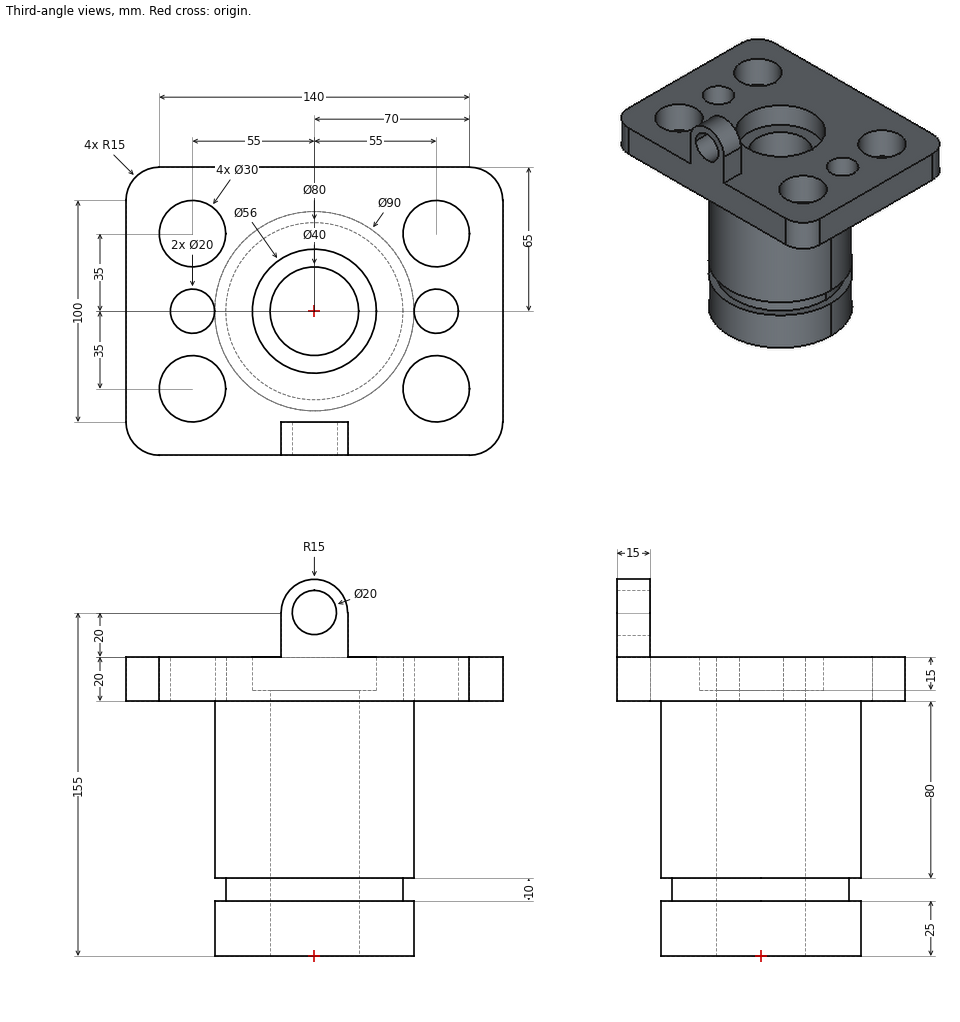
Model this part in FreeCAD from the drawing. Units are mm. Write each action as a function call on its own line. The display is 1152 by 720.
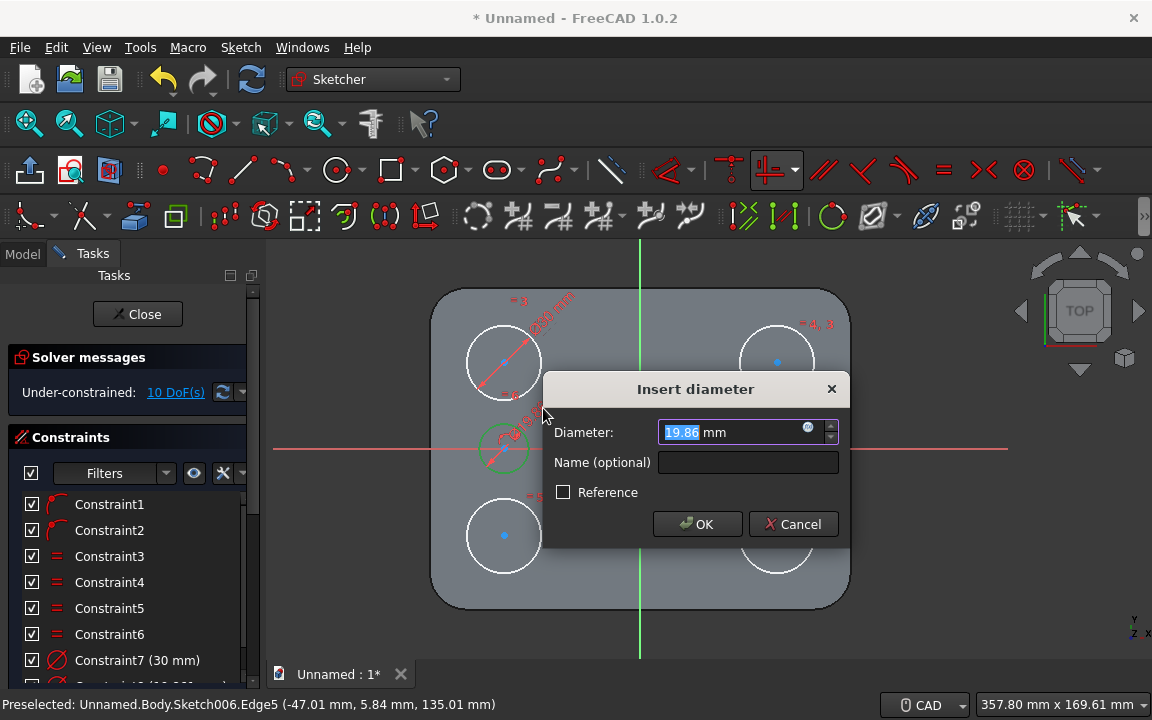
text(20)
key(Return)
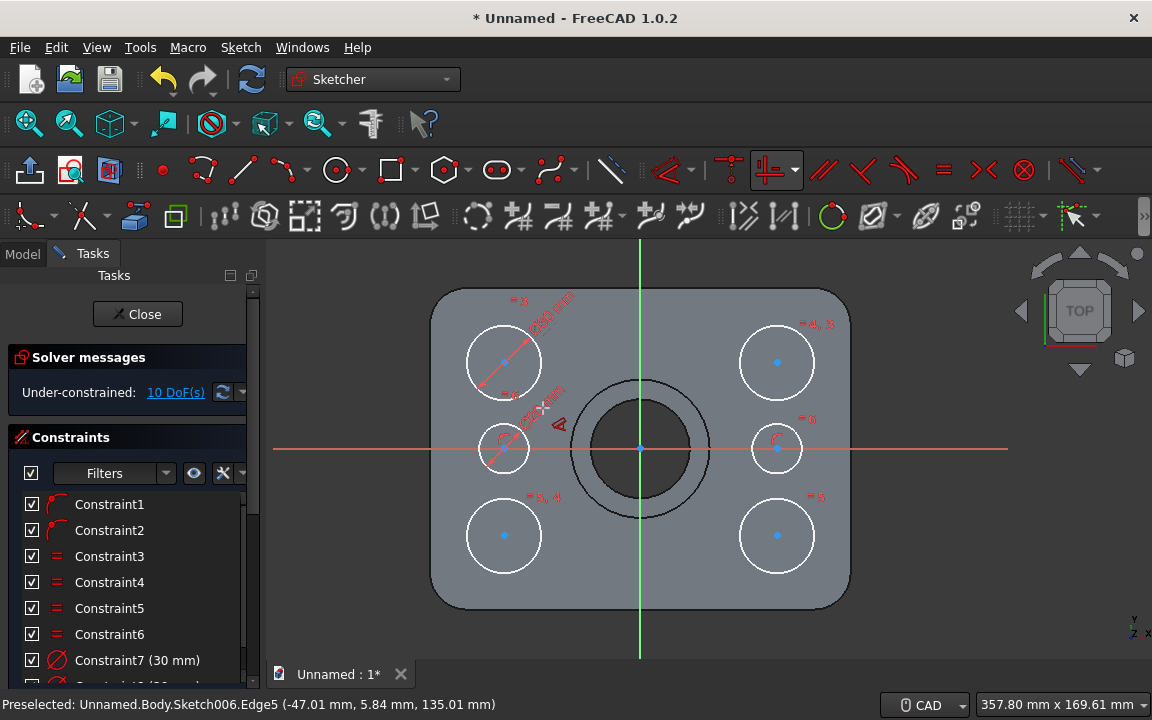
click(504, 363)
click(572, 483)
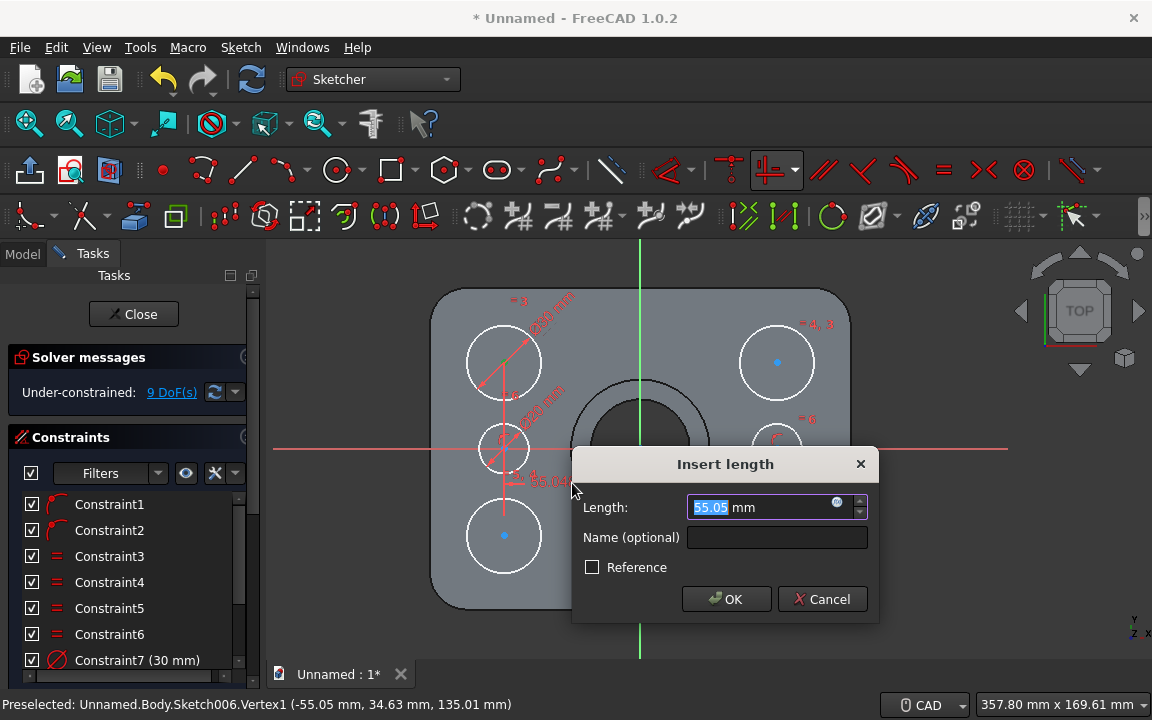
text(55)
key(Return)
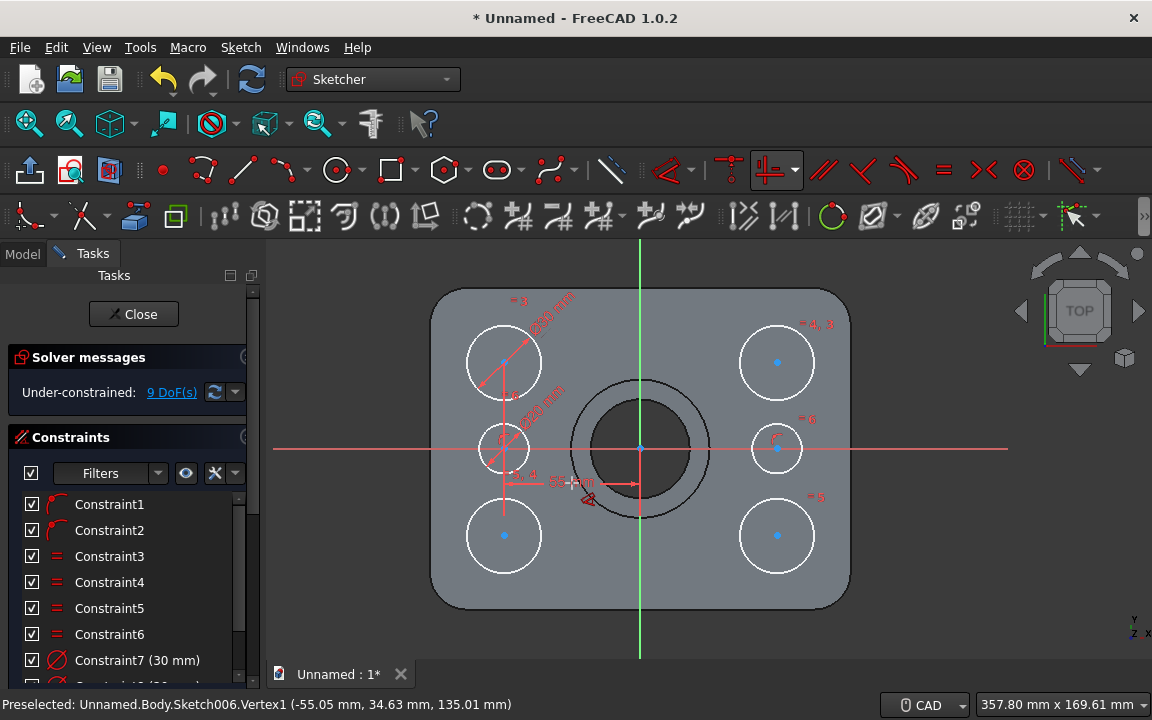
click(504, 363)
click(470, 406)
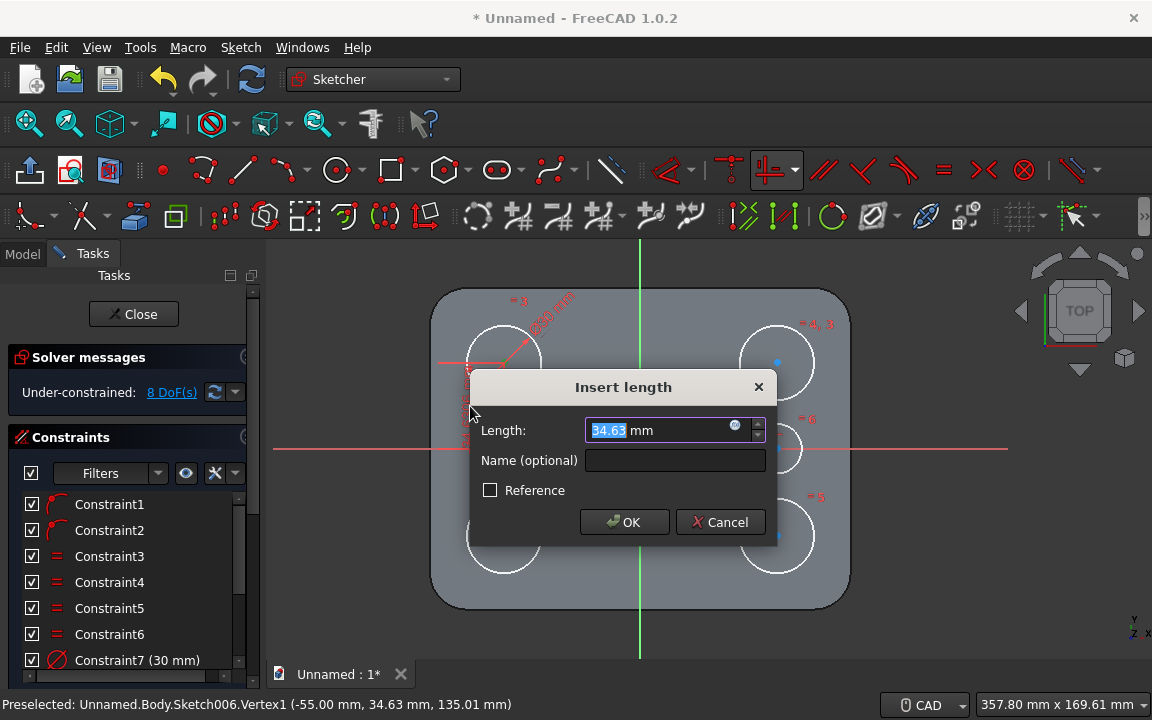
text(35)
key(Return)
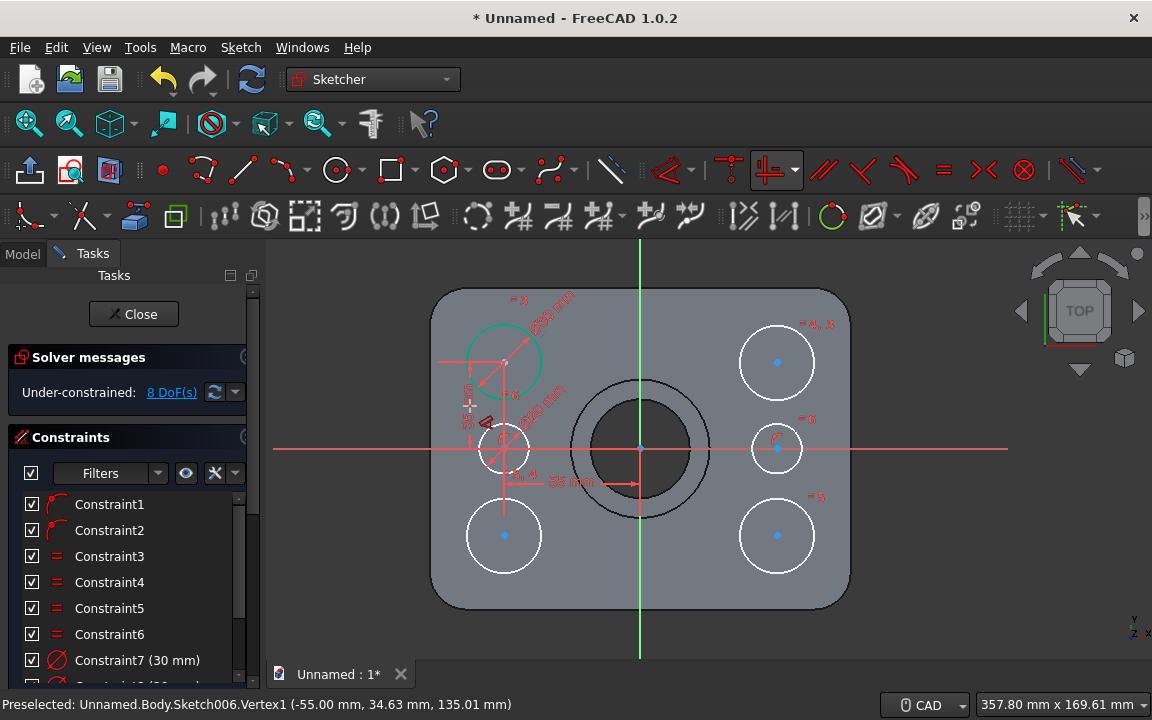
click(777, 363)
click(709, 329)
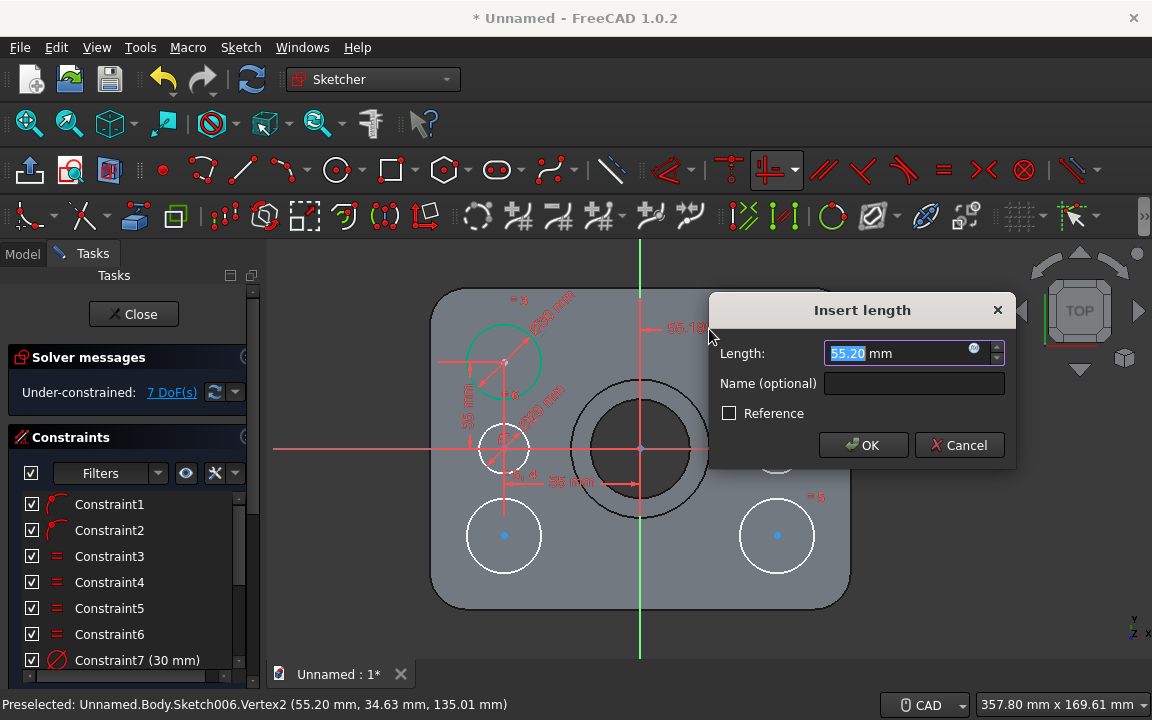
text(55)
key(Return)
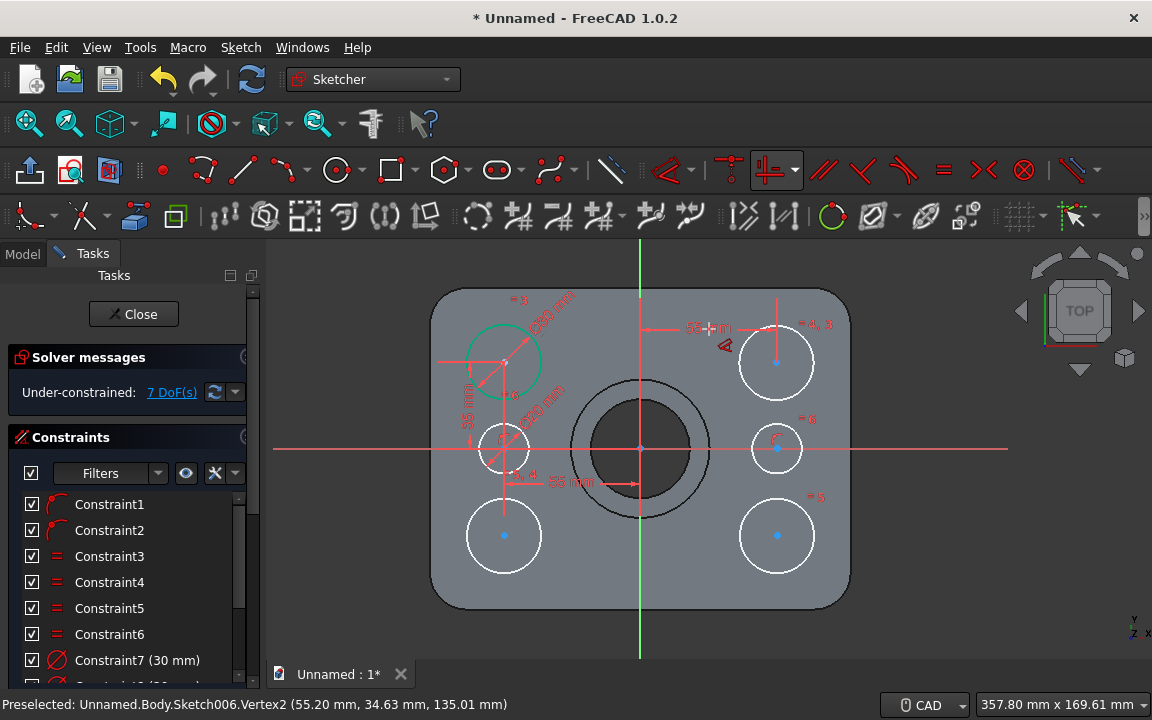
click(777, 363)
click(811, 406)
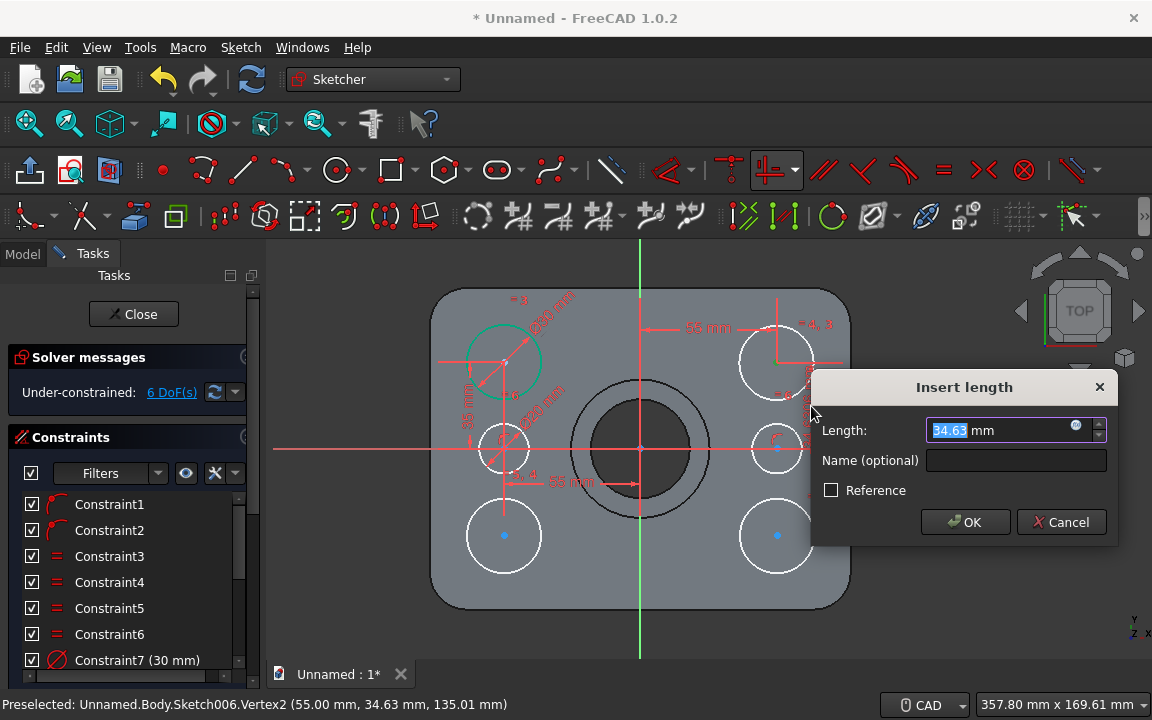
text(35)
key(Return)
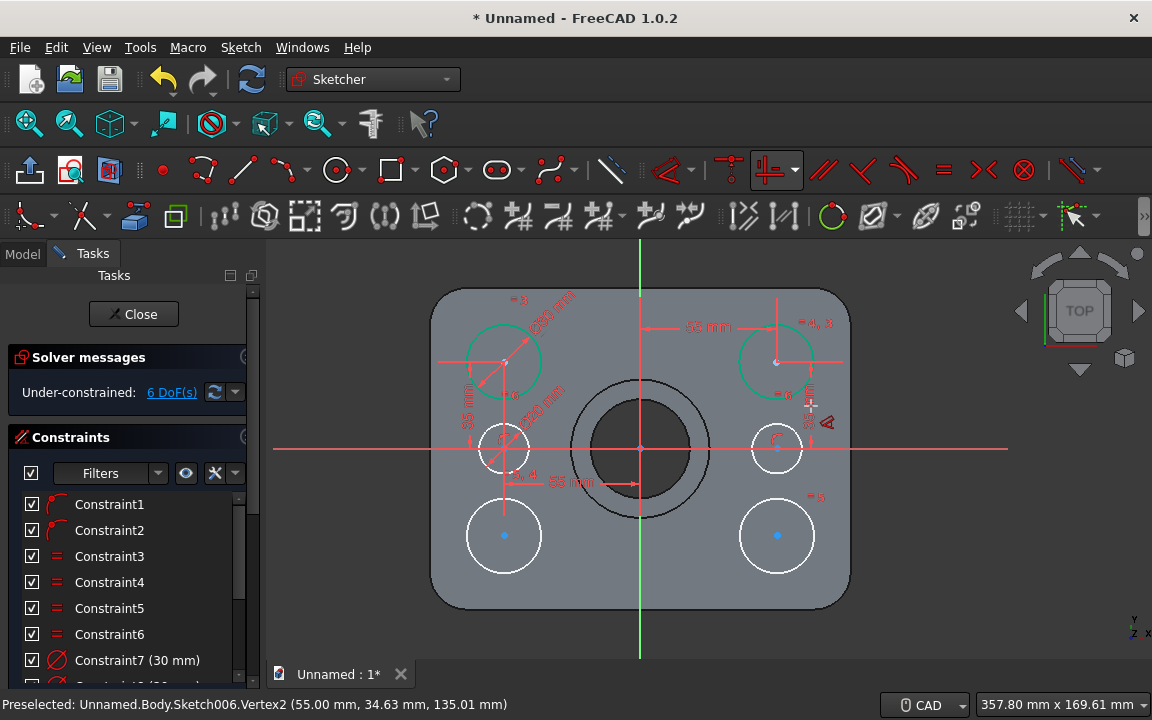
click(504, 536)
click(572, 570)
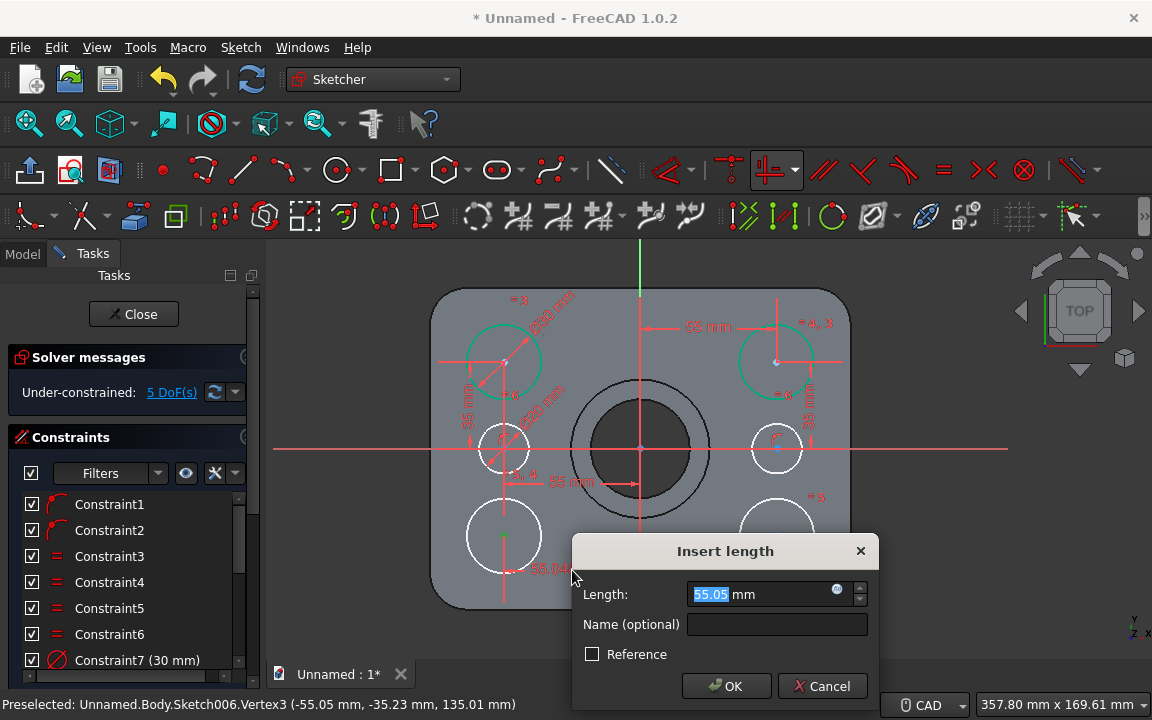
text(55)
key(Return)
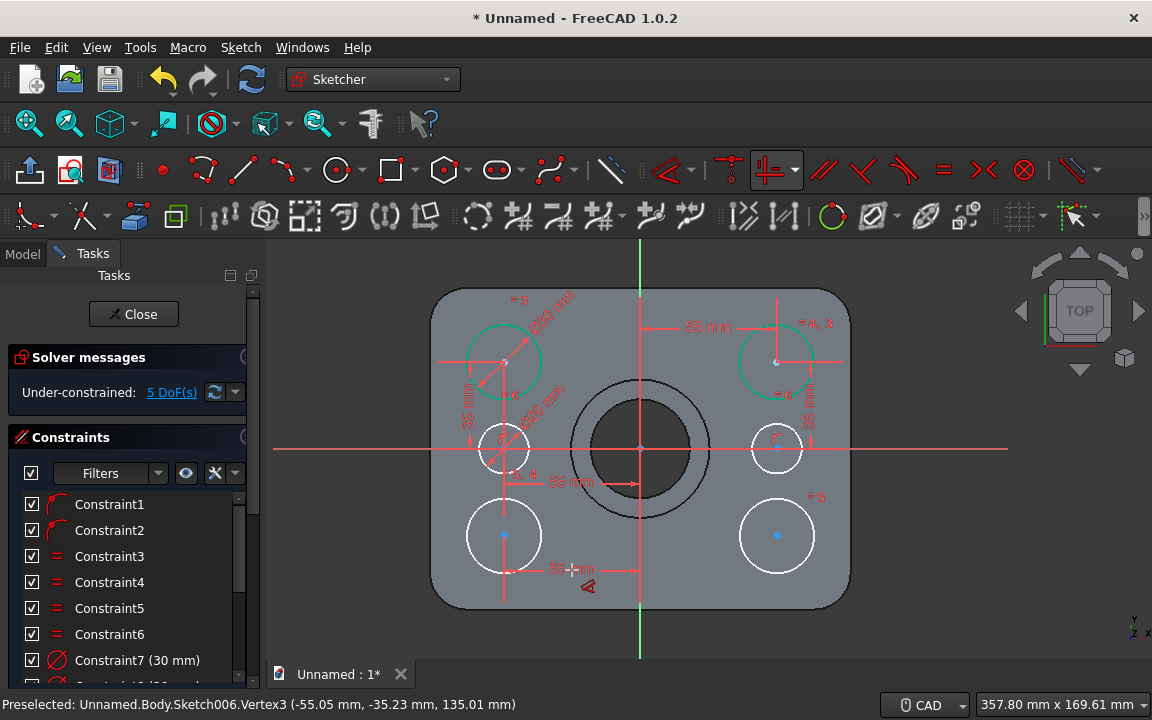
click(504, 536)
click(470, 492)